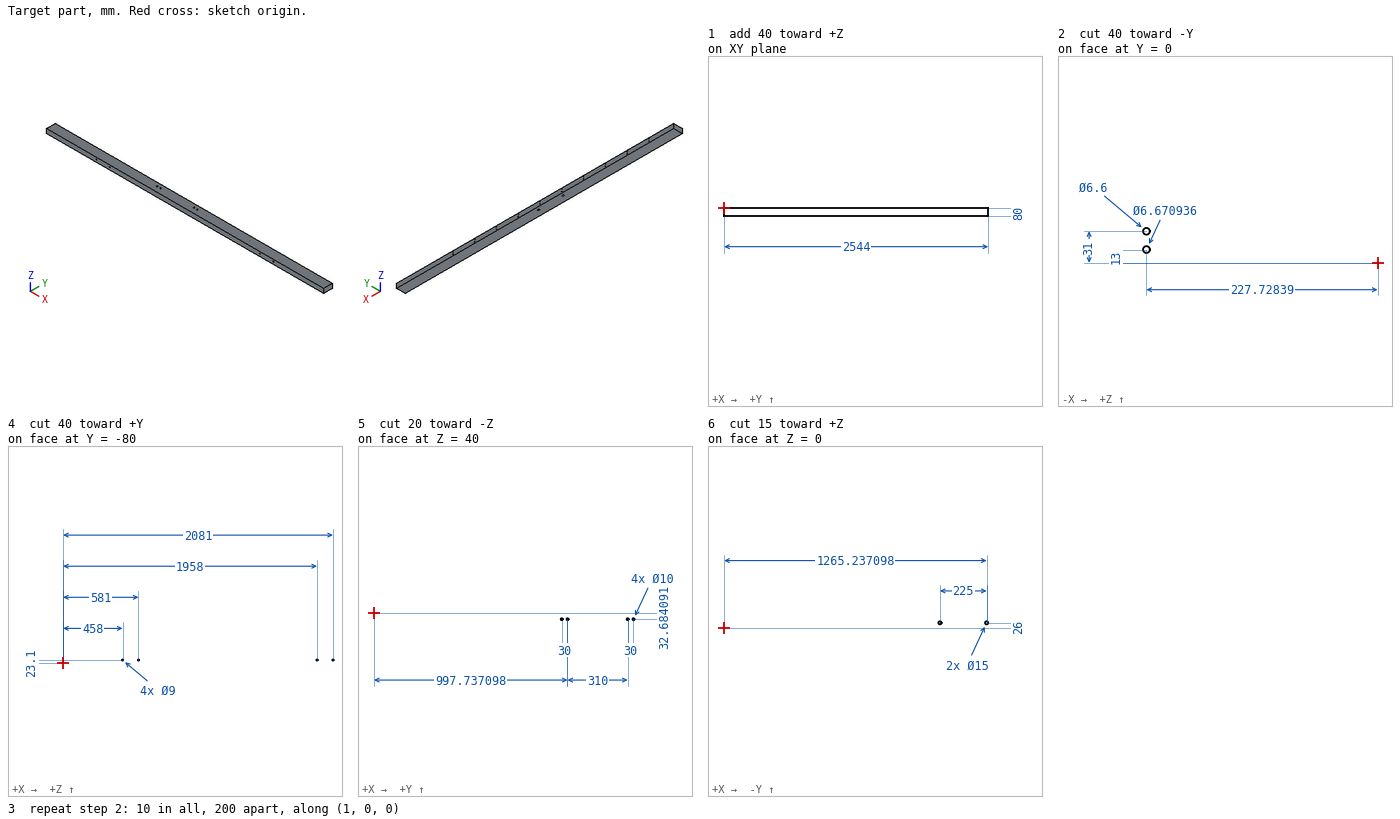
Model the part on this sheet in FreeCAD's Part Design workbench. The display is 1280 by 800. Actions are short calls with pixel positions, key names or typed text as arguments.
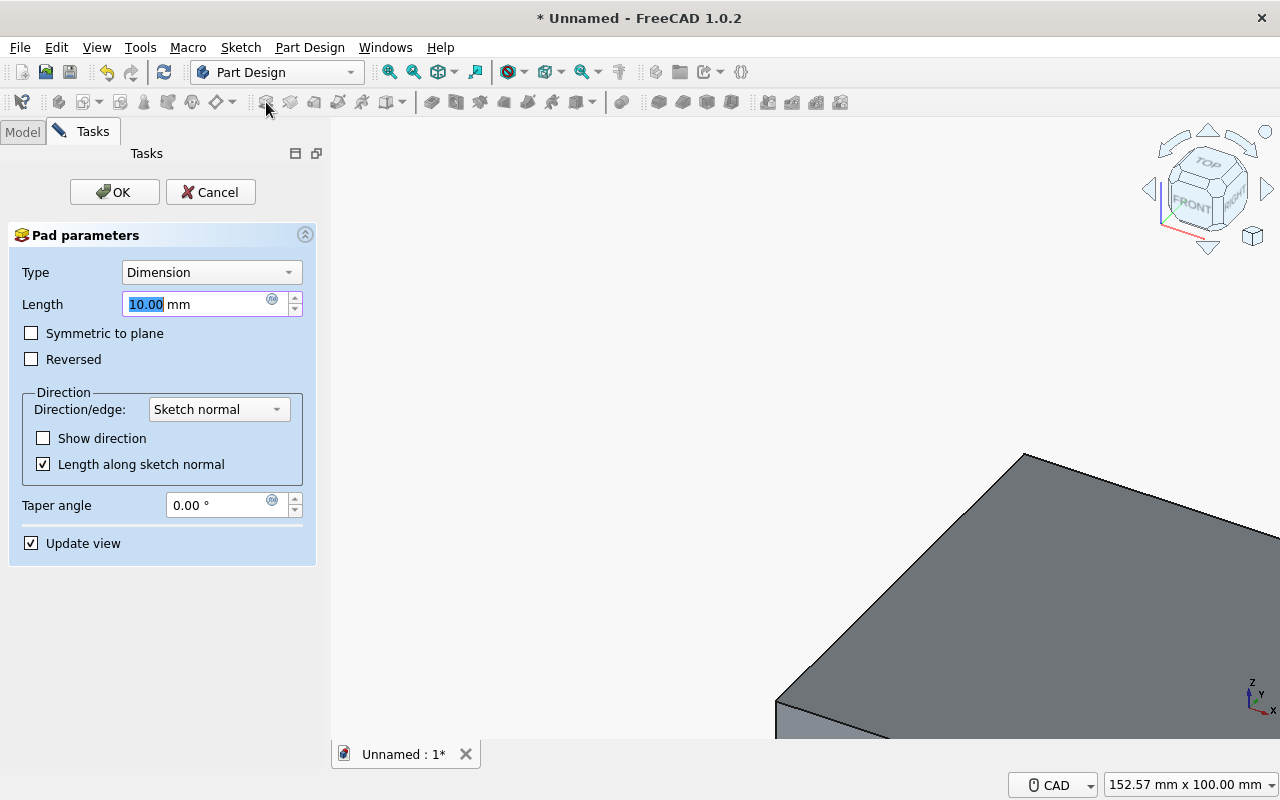
text(40)
key(Tab)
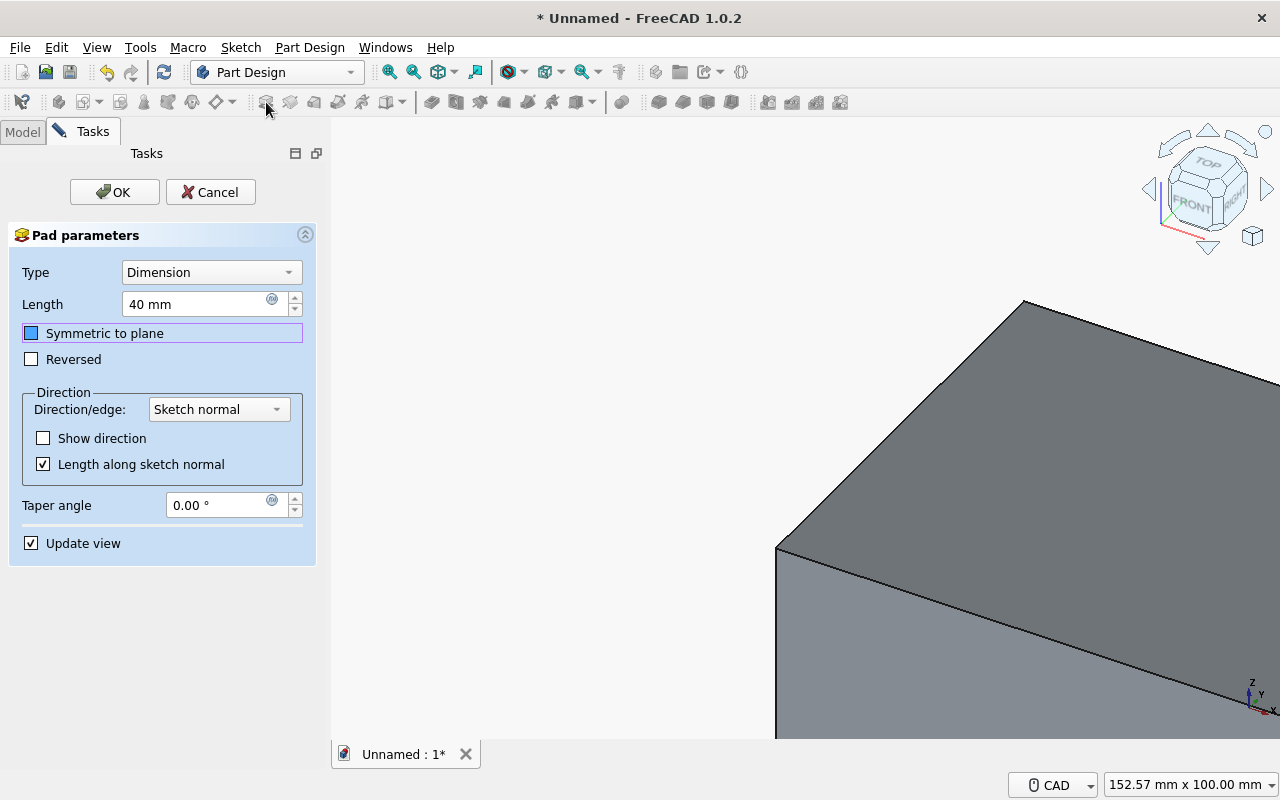
click(115, 192)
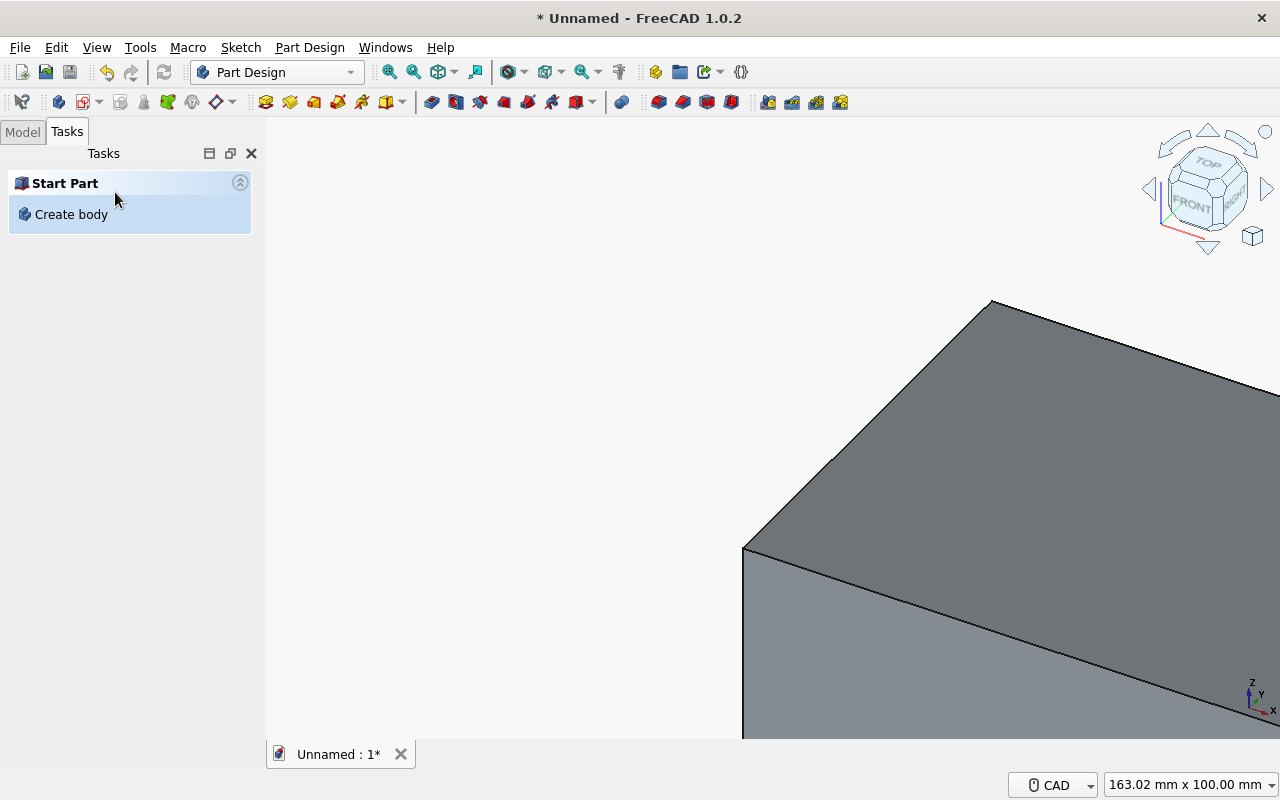
key(v)
key(f)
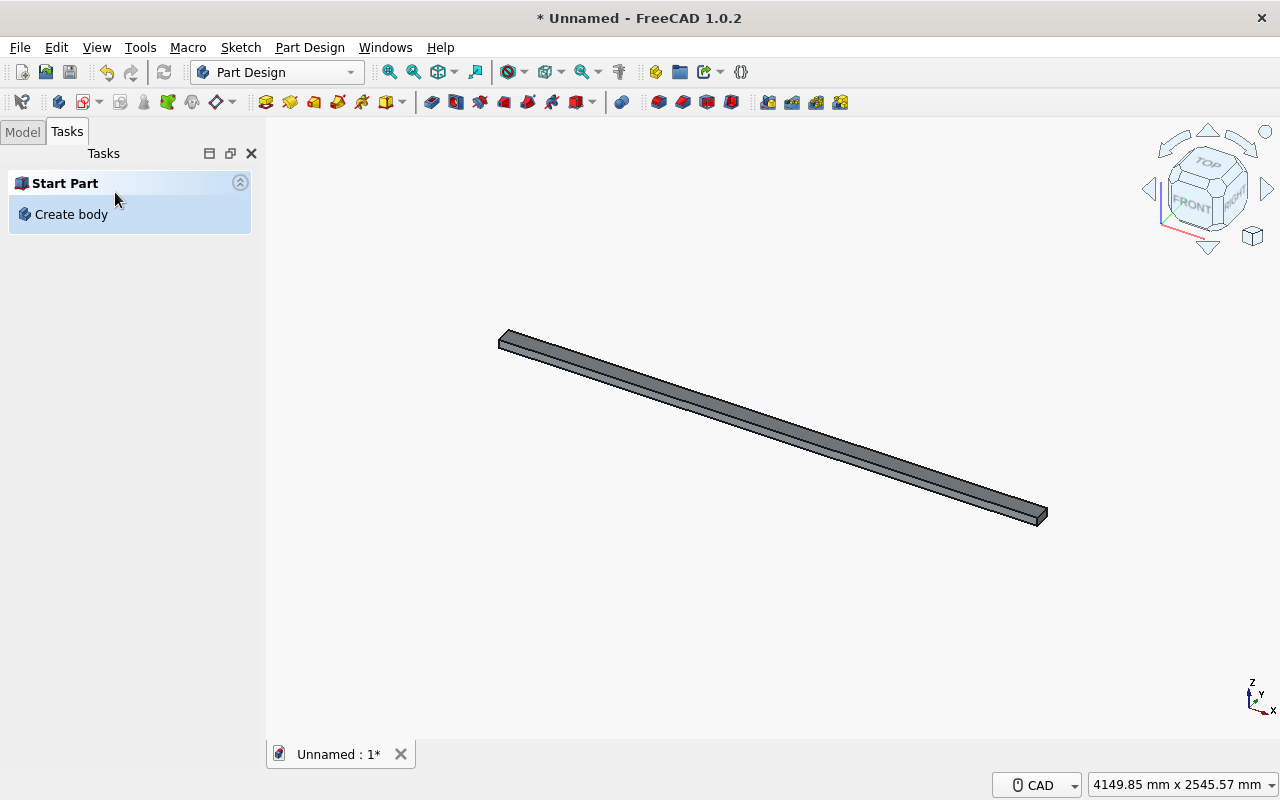
key(4)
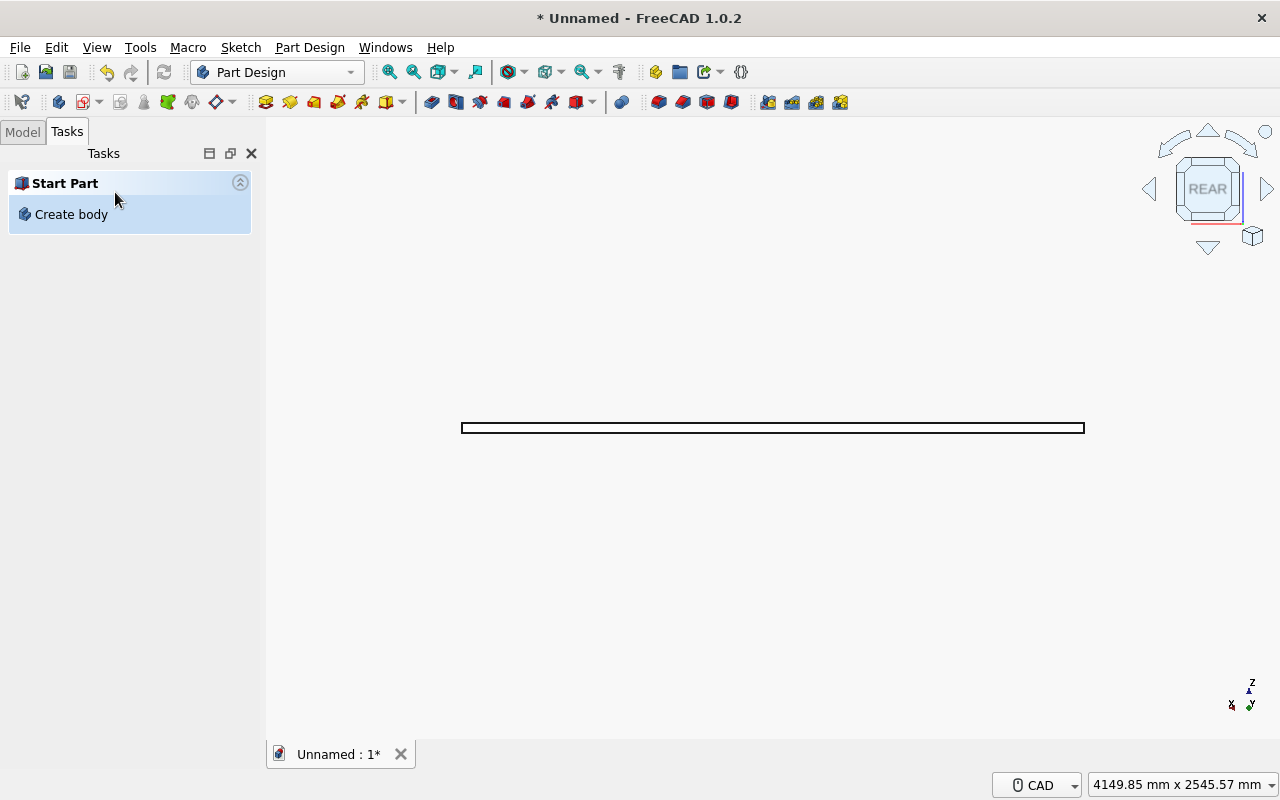
scroll(507, 427, up, 5)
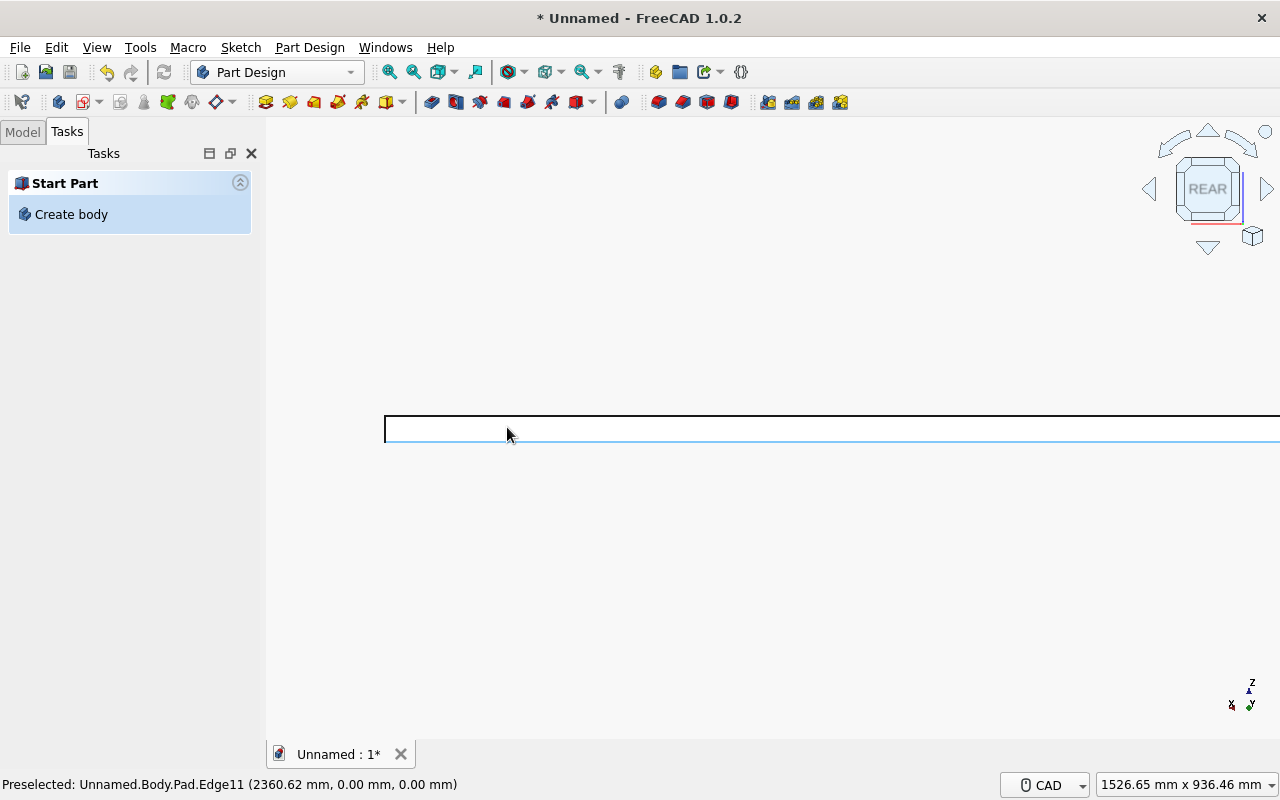
click(505, 428)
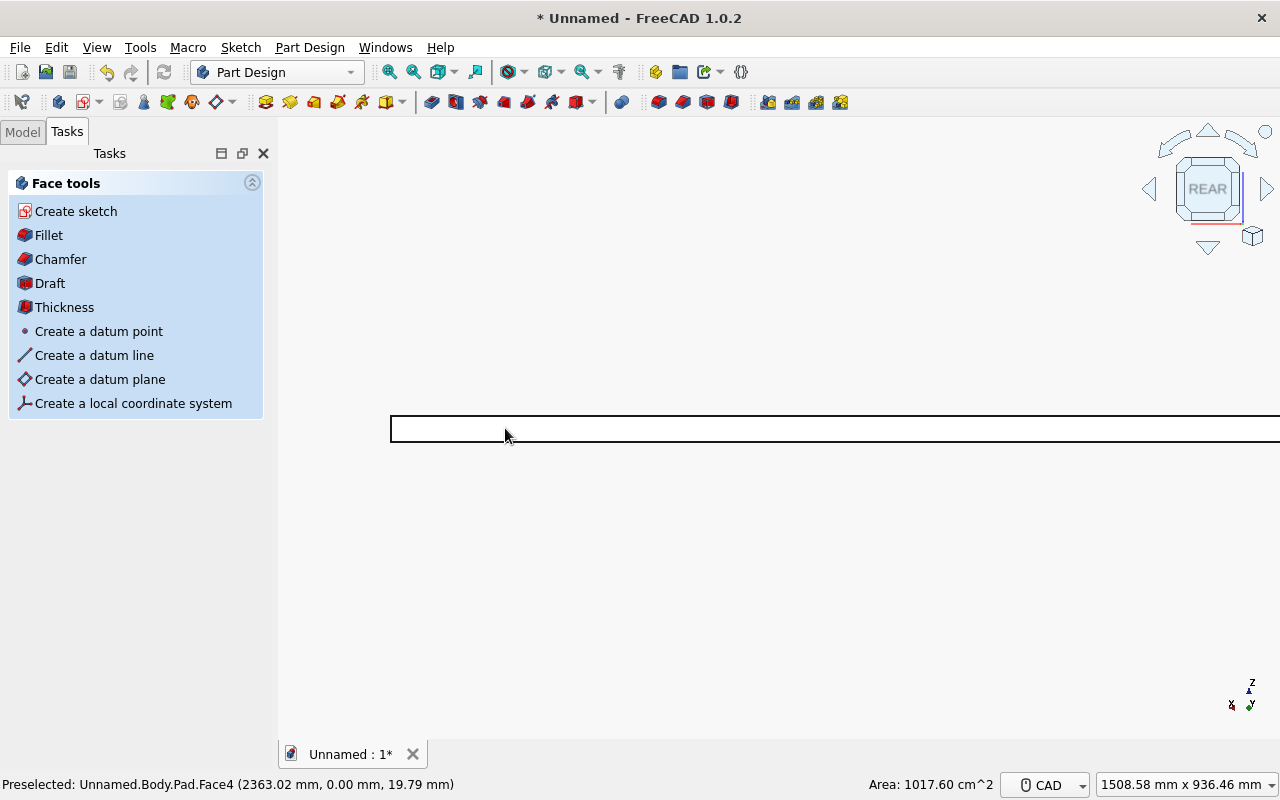
click(84, 102)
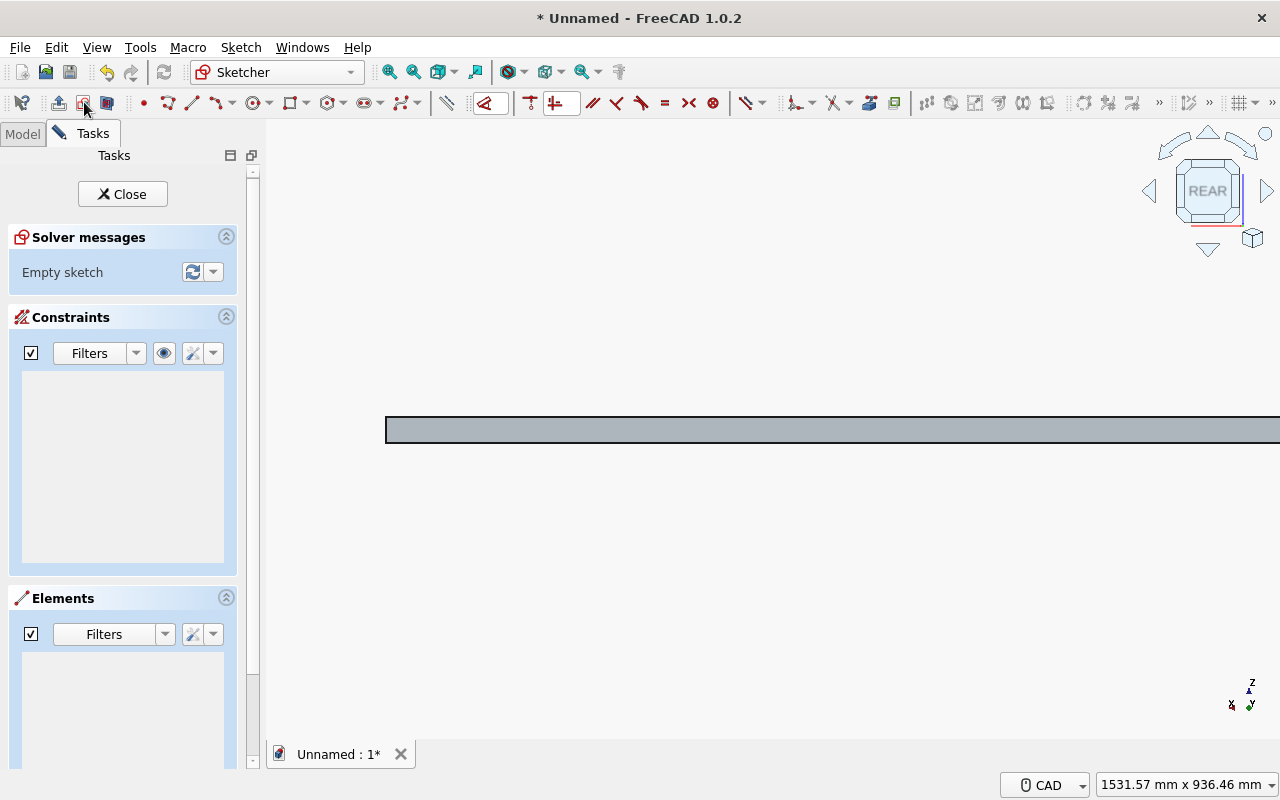
scroll(704, 429, down, 5)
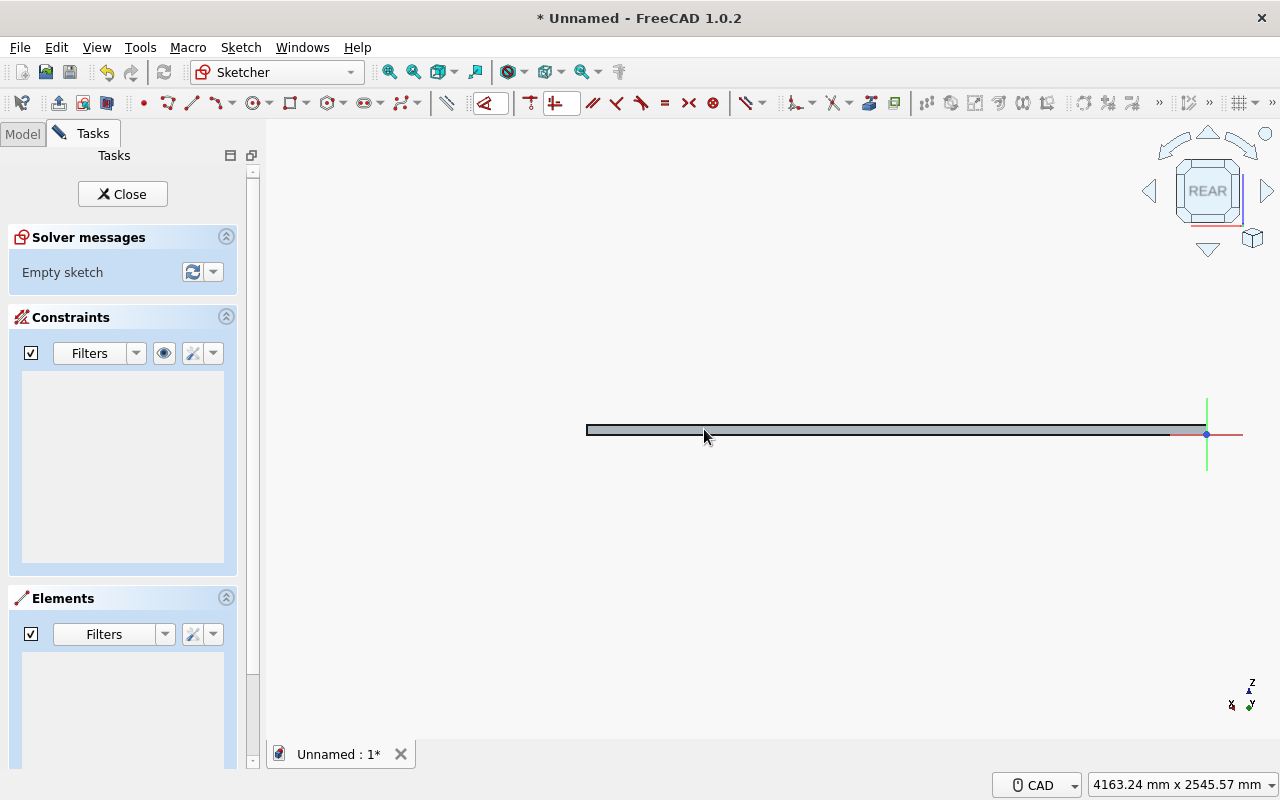
scroll(704, 429, down, 5)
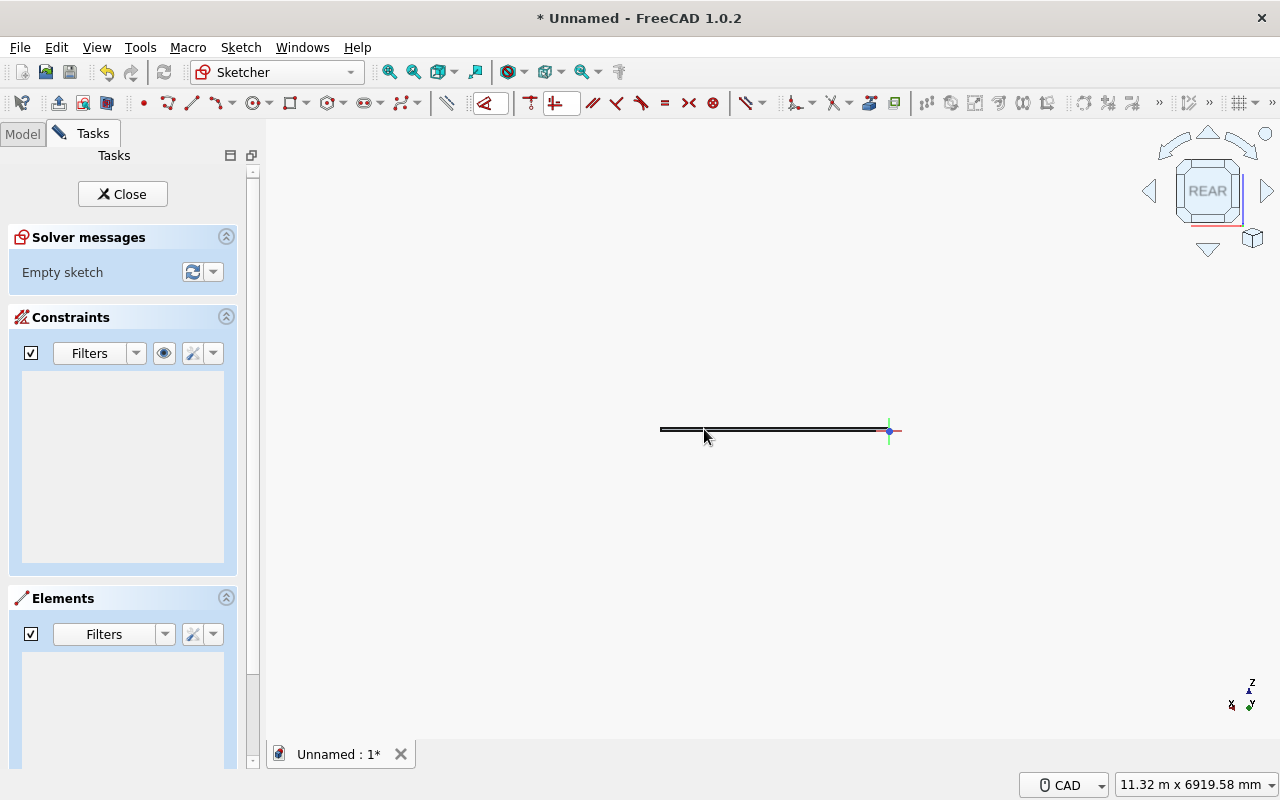
scroll(877, 429, up, 15)